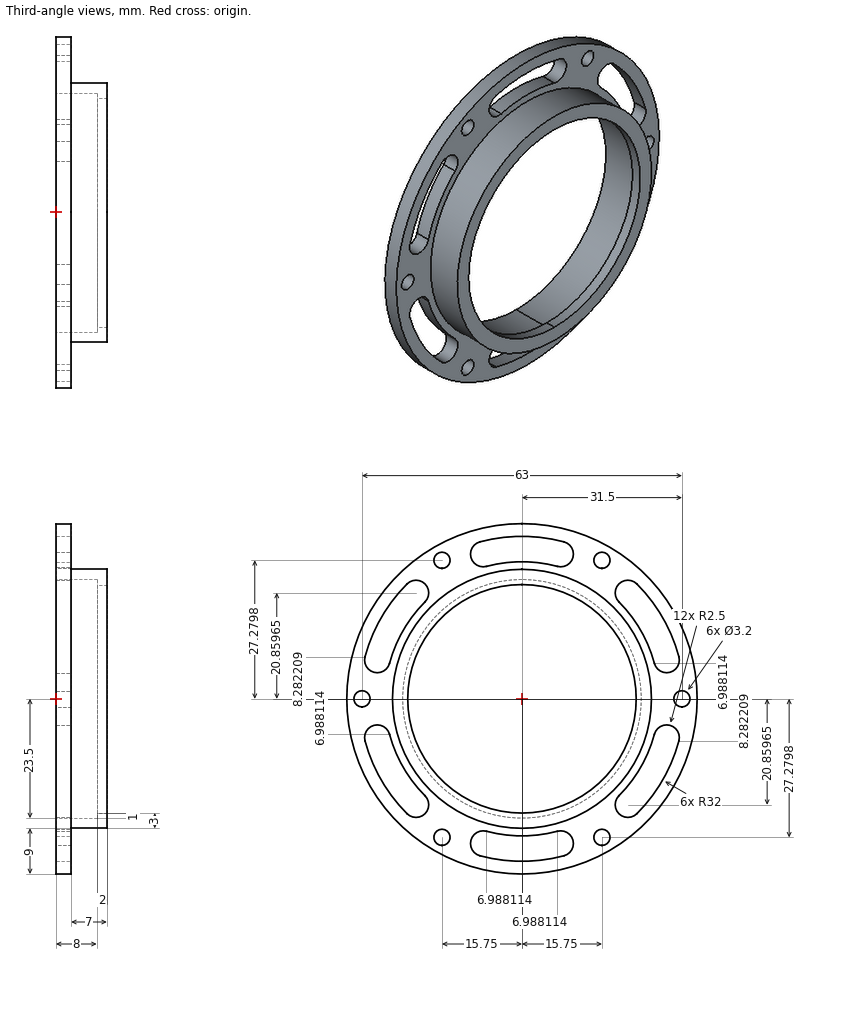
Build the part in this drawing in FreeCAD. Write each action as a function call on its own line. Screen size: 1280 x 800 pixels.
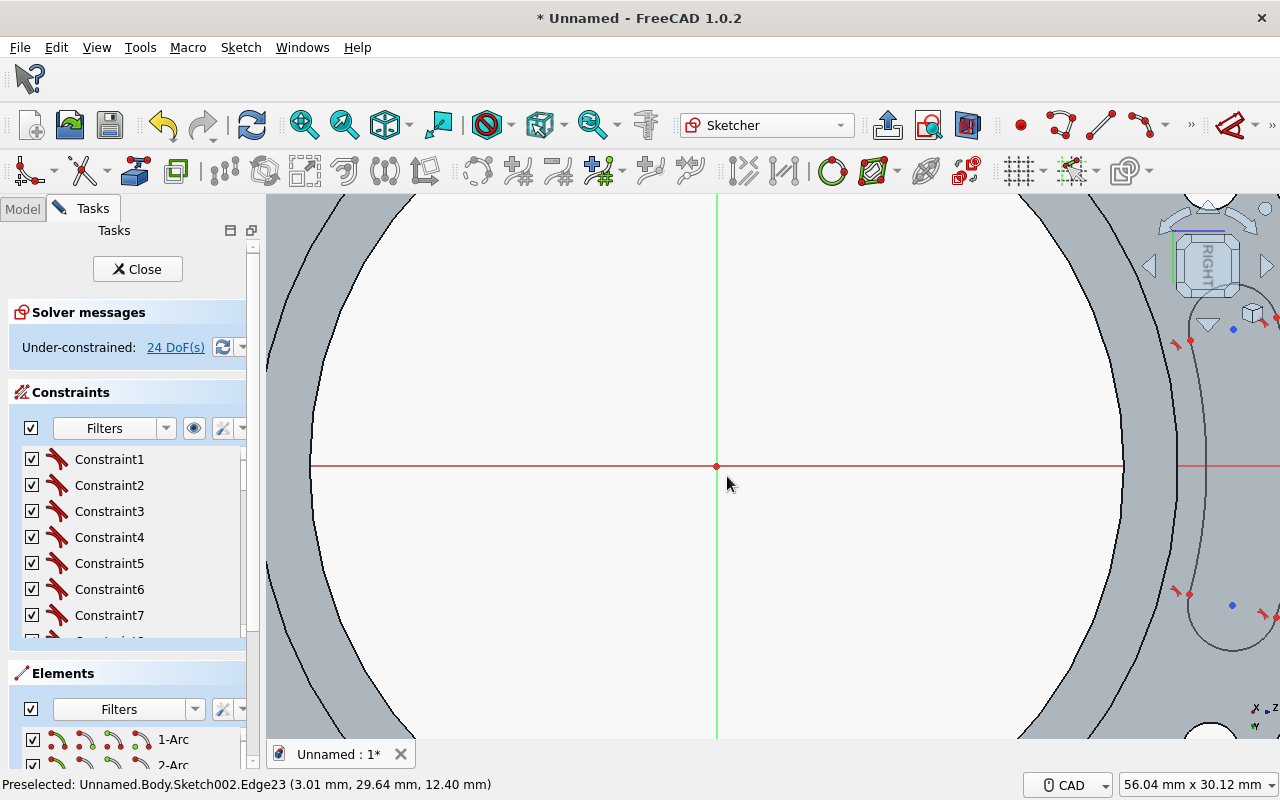
scroll(699, 467, down, 6)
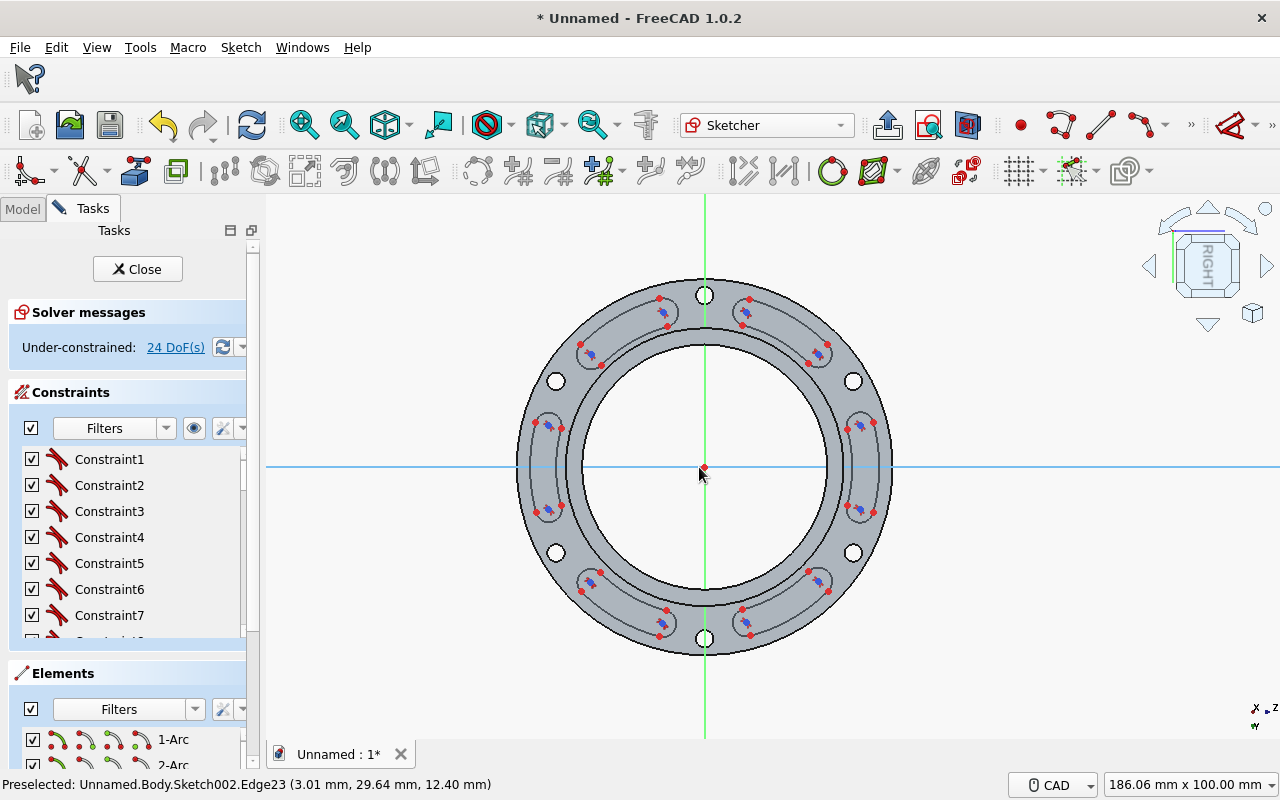
click(618, 588)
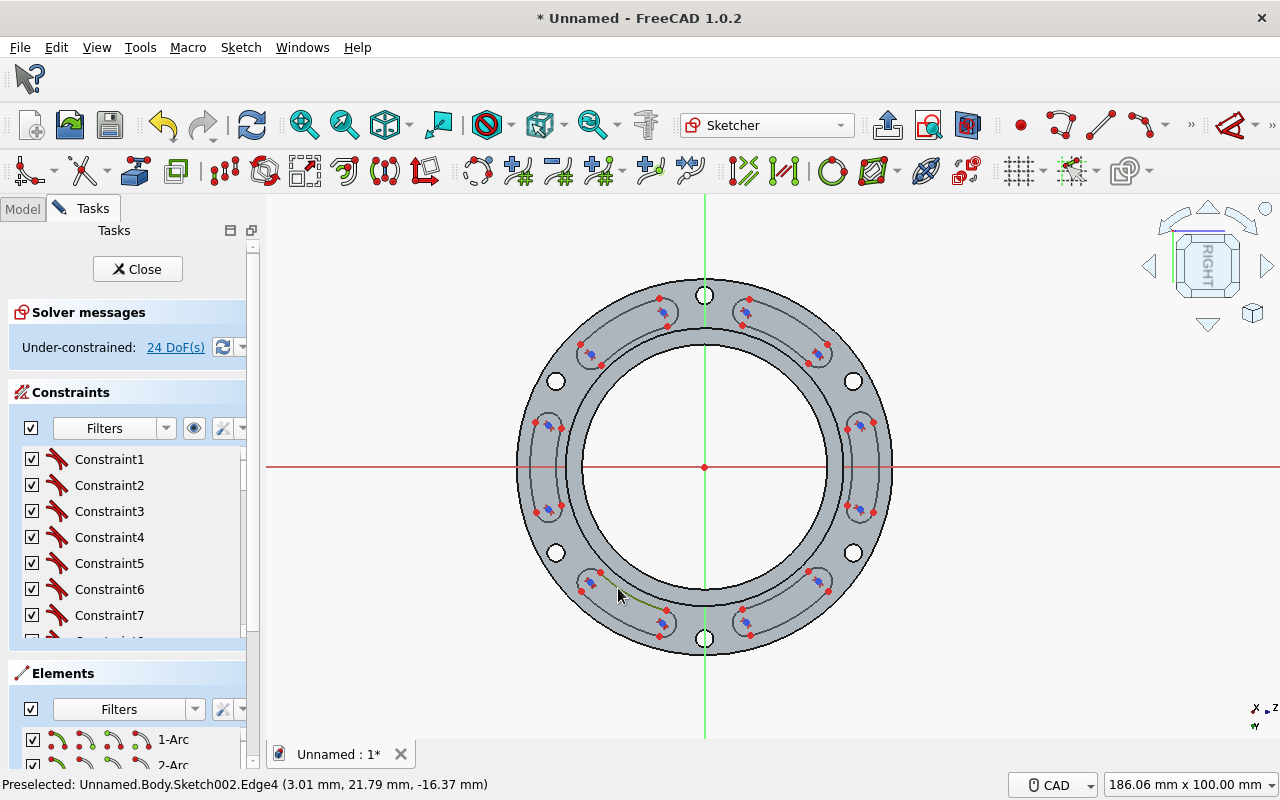
click(557, 452)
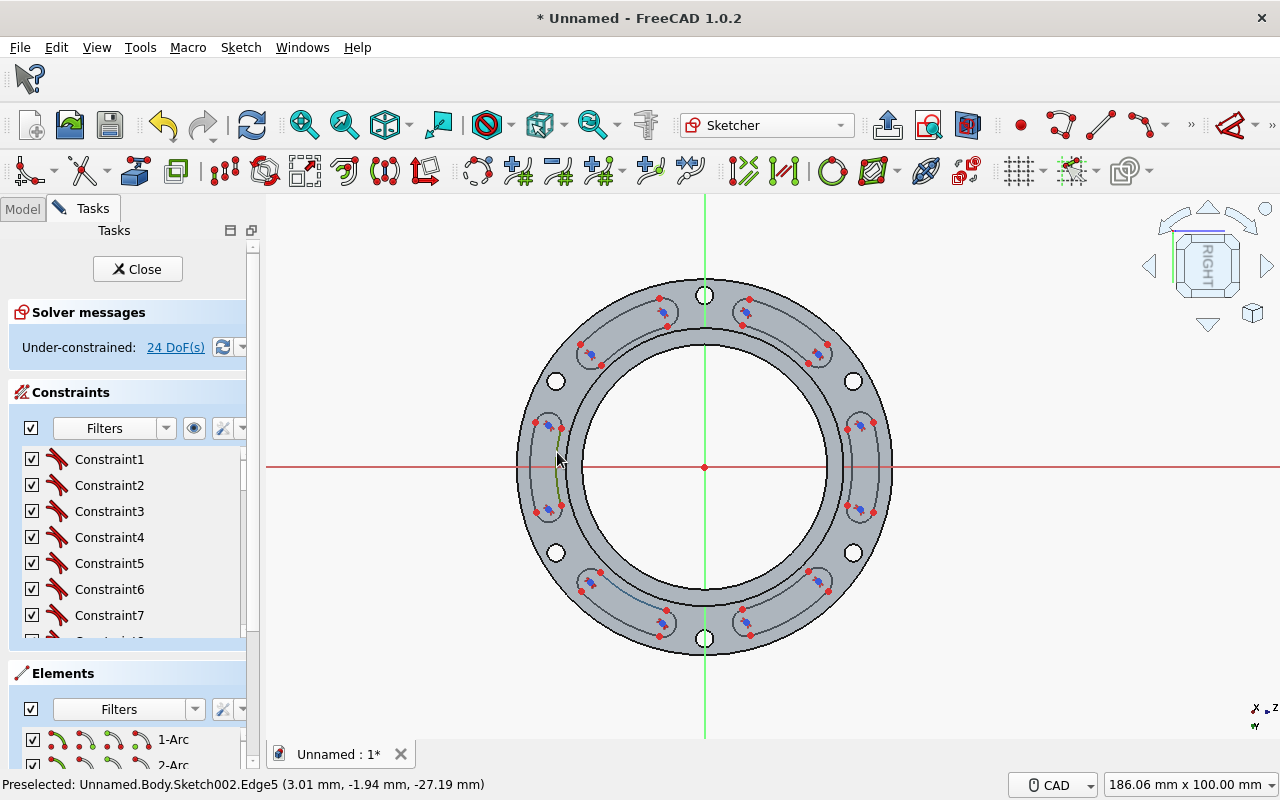
click(646, 335)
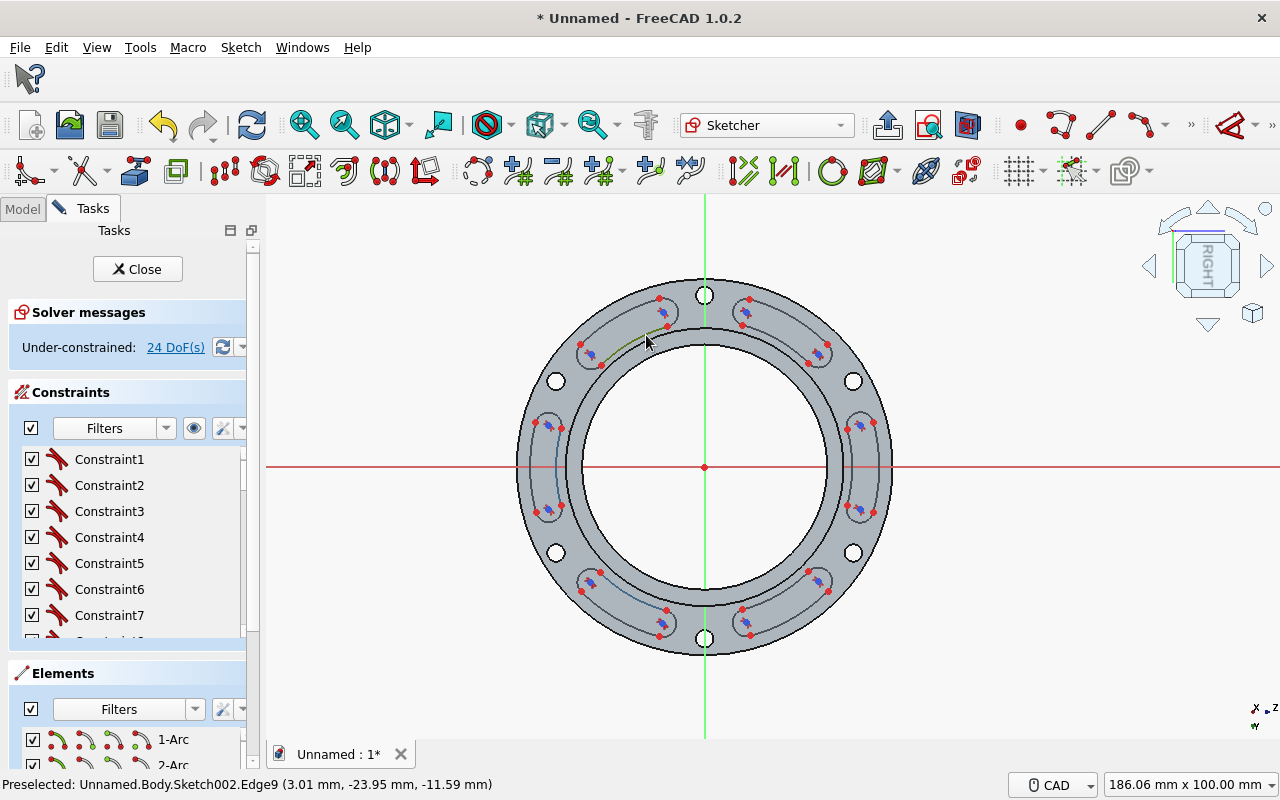
click(791, 348)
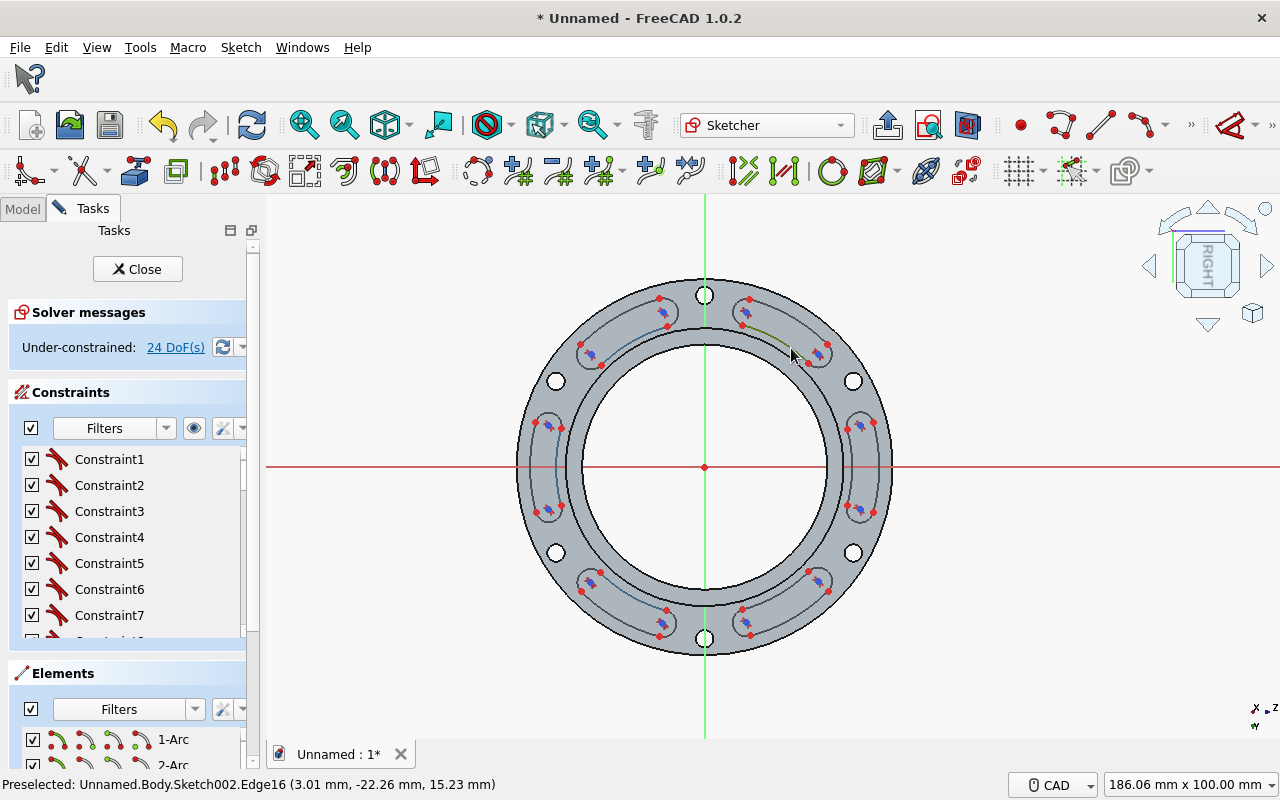
click(851, 483)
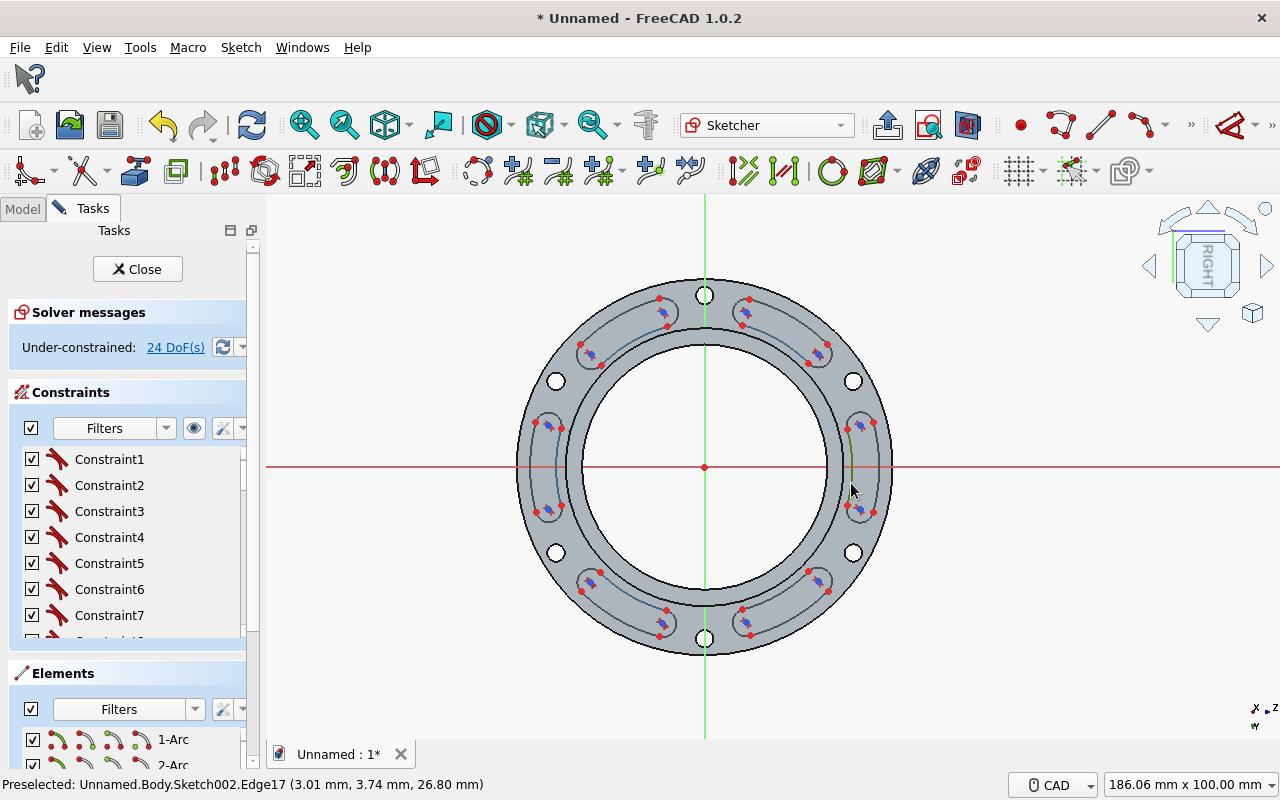
click(765, 602)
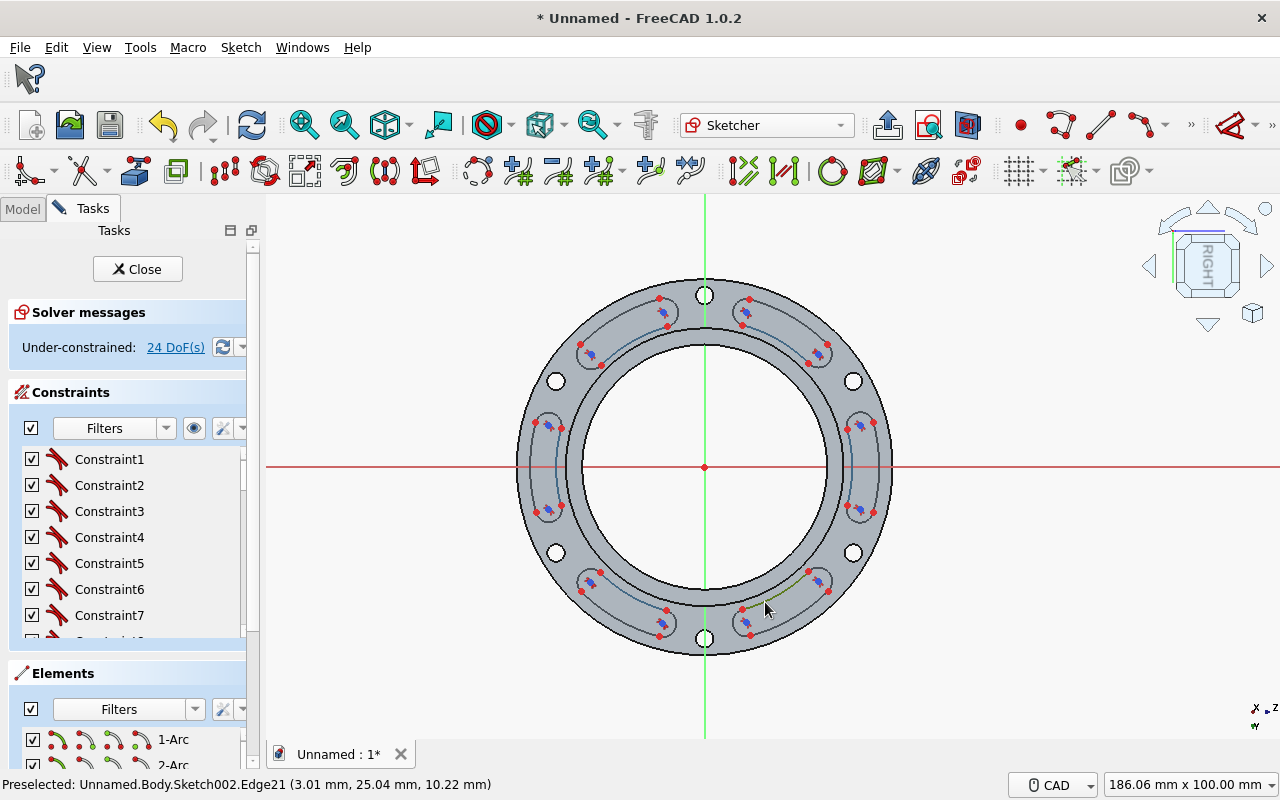
key(e)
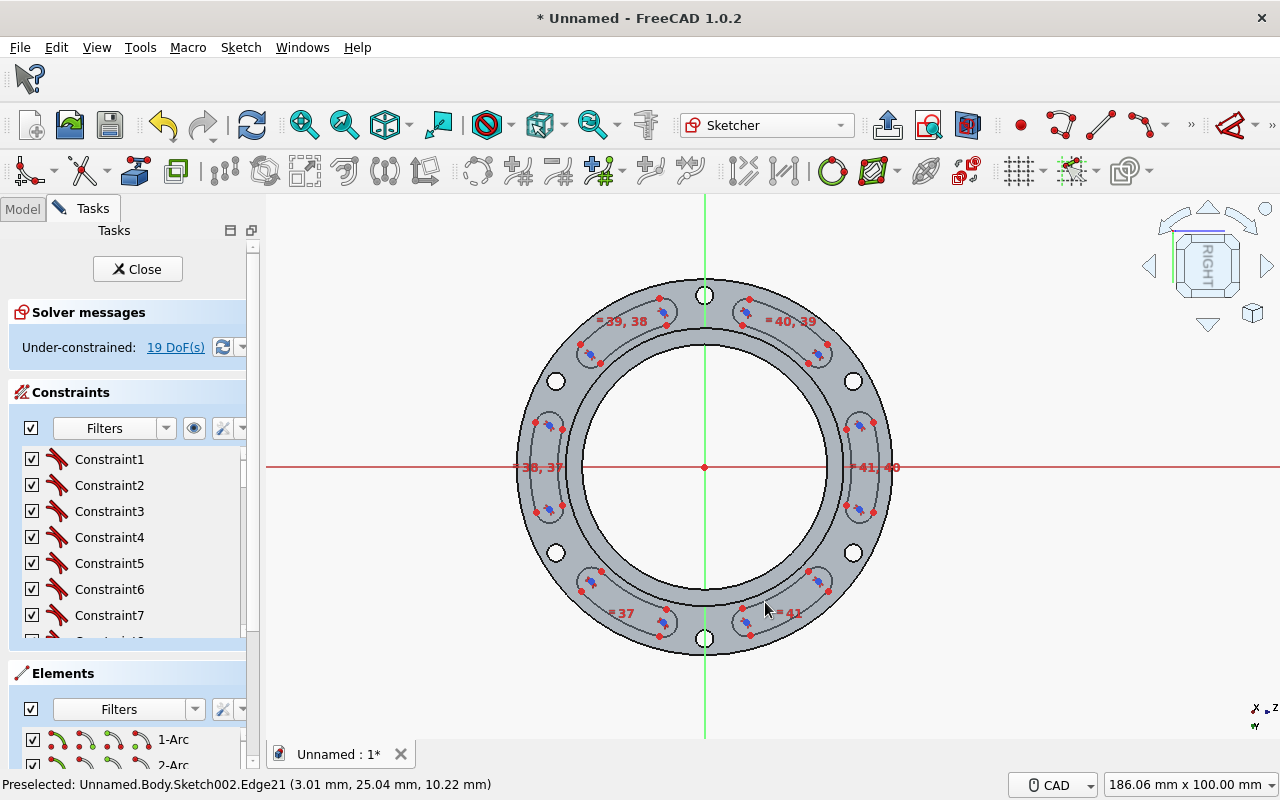
click(589, 568)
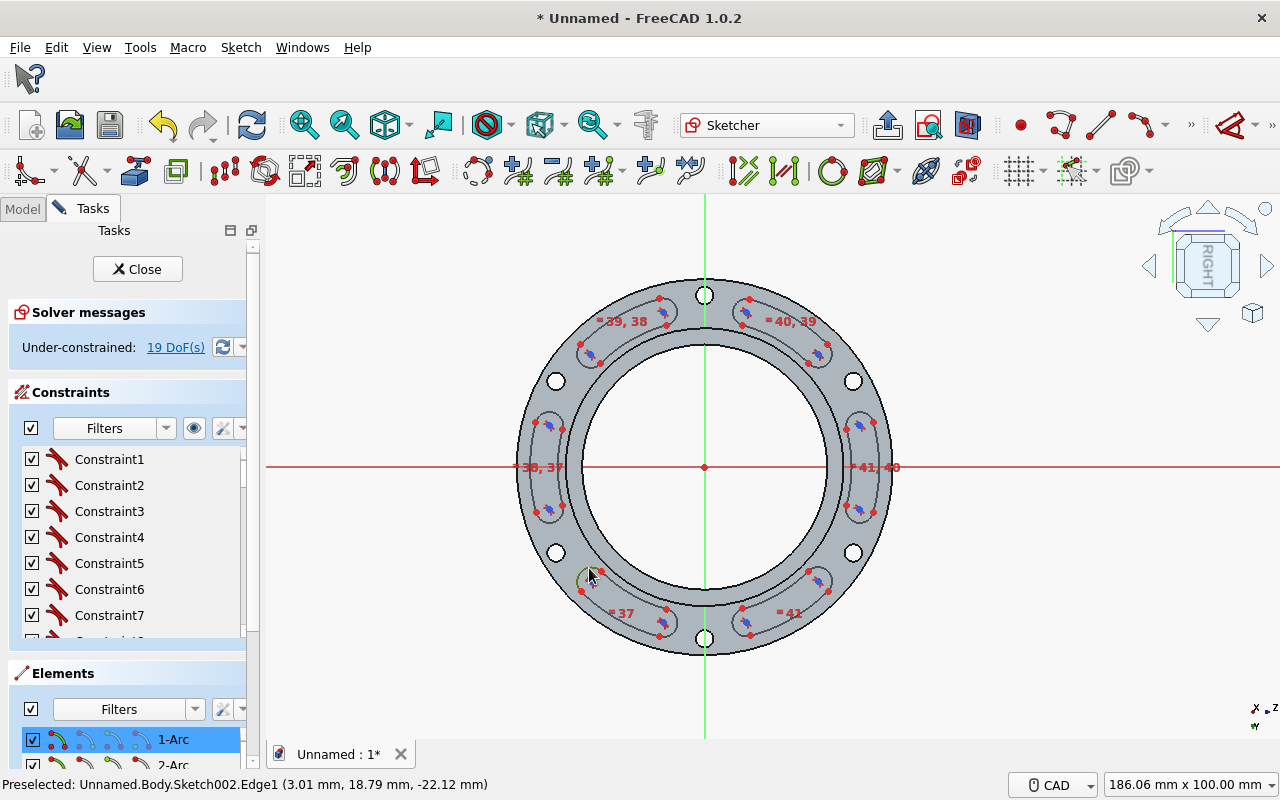
click(560, 417)